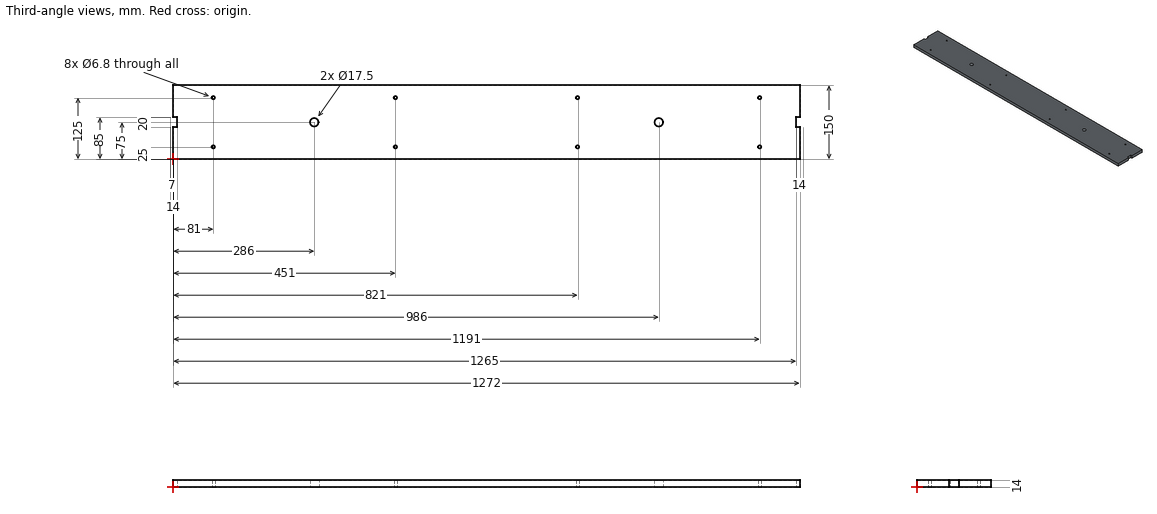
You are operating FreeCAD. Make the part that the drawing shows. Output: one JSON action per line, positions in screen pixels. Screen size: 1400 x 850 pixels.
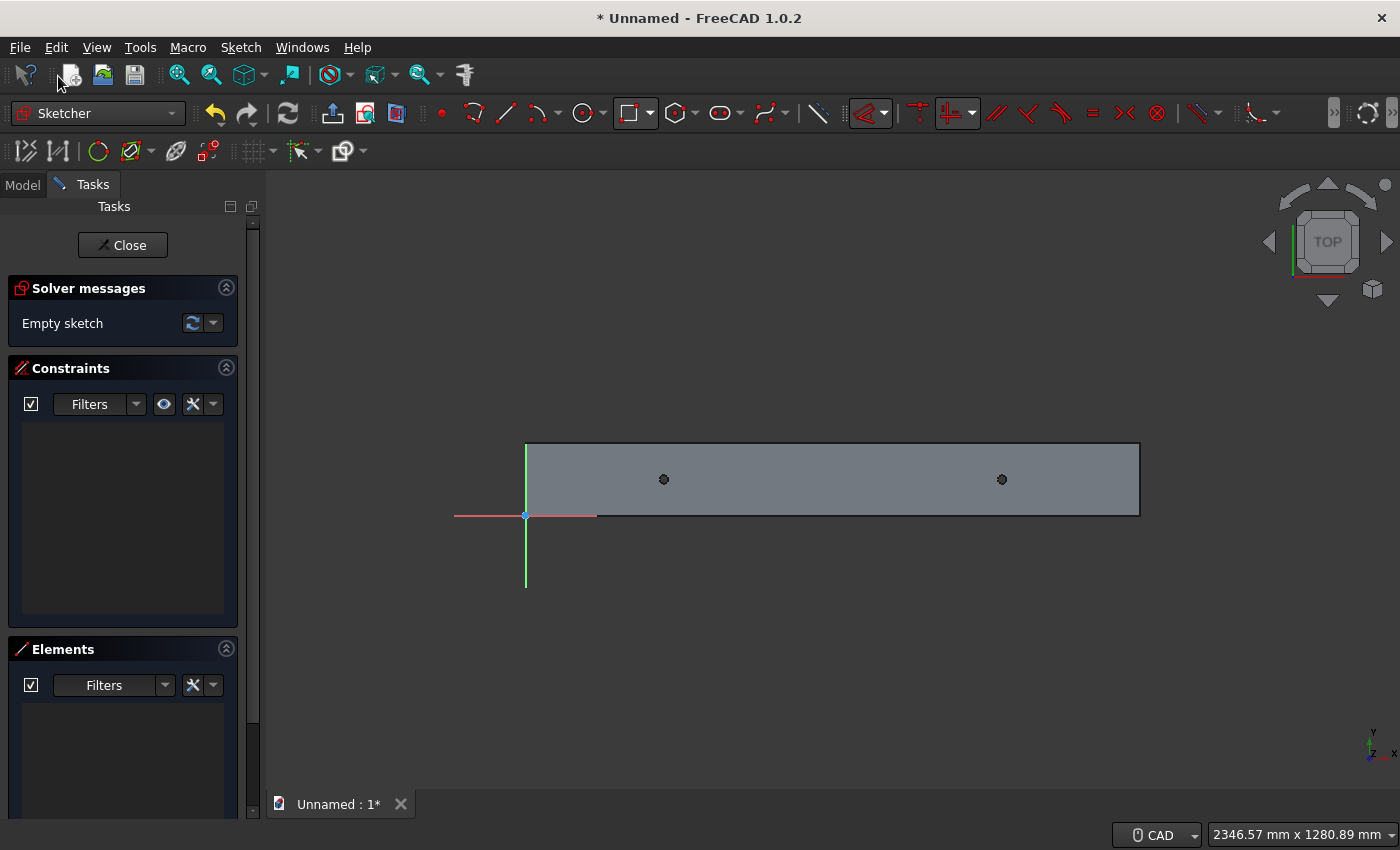
{"action": "left_click", "coordinate": [584, 114]}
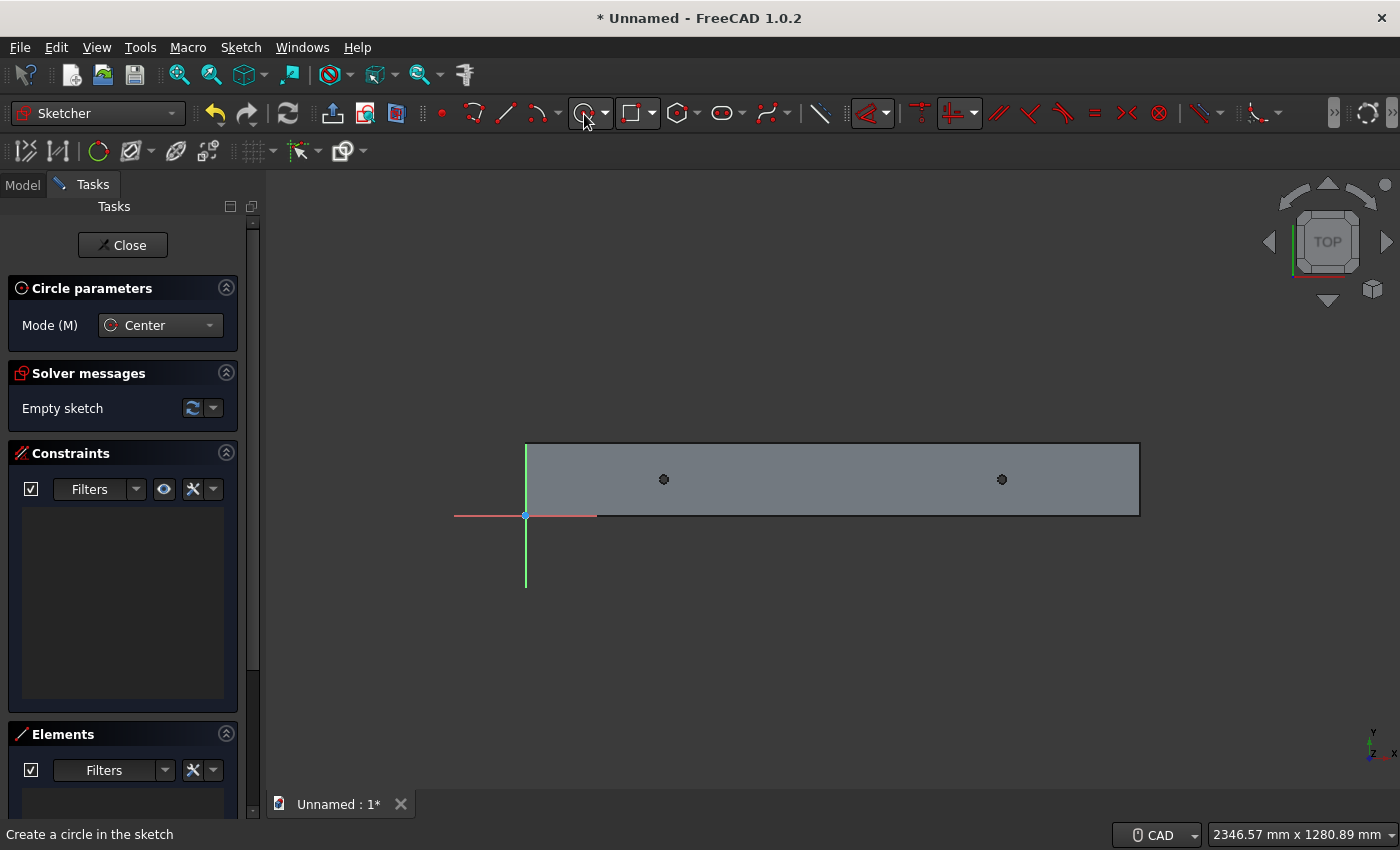
{"action": "scroll", "coordinate": [565, 455], "scroll_direction": "up", "scroll_amount": 14}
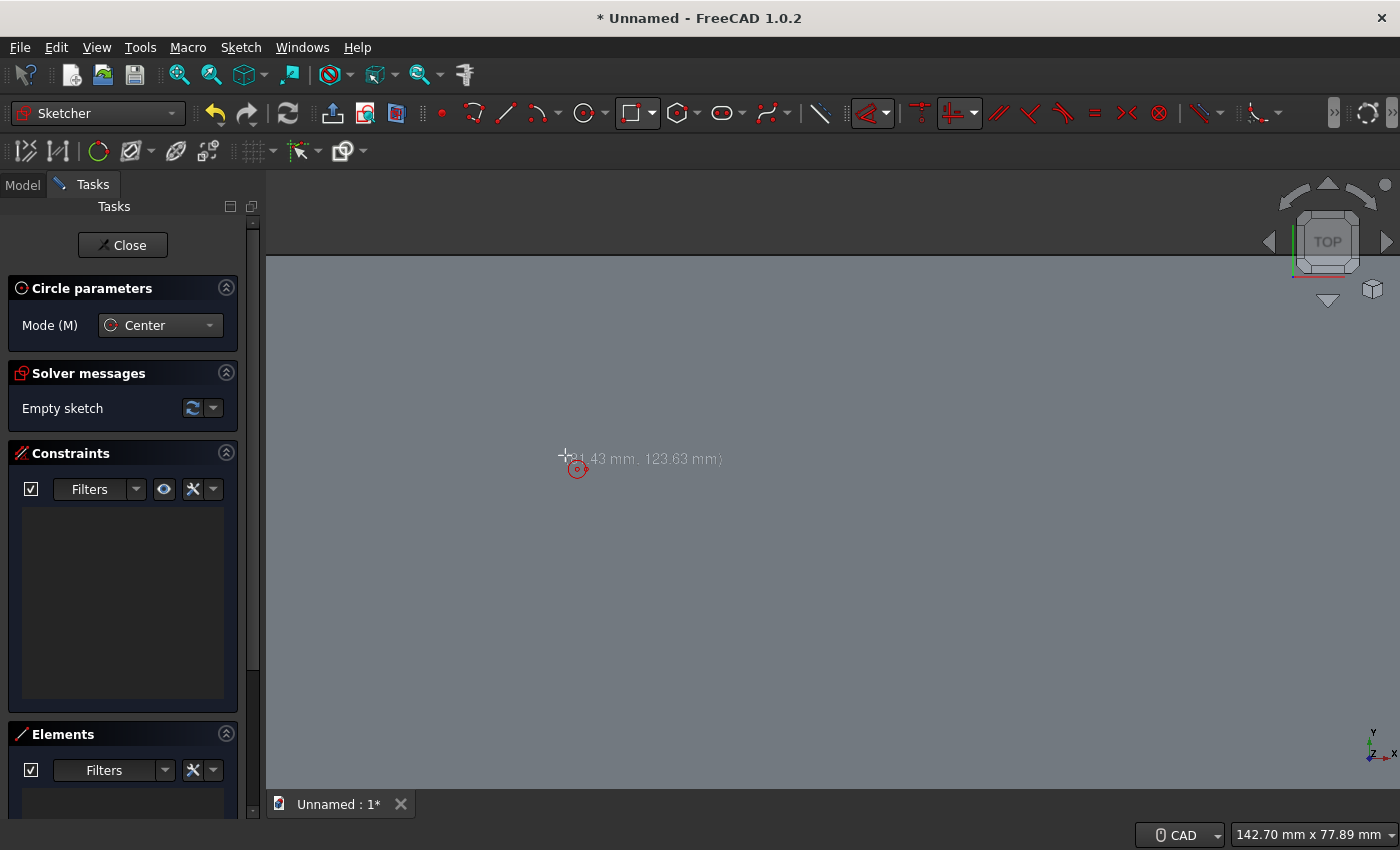
{"action": "scroll", "coordinate": [452, 443], "scroll_direction": "down", "scroll_amount": 13}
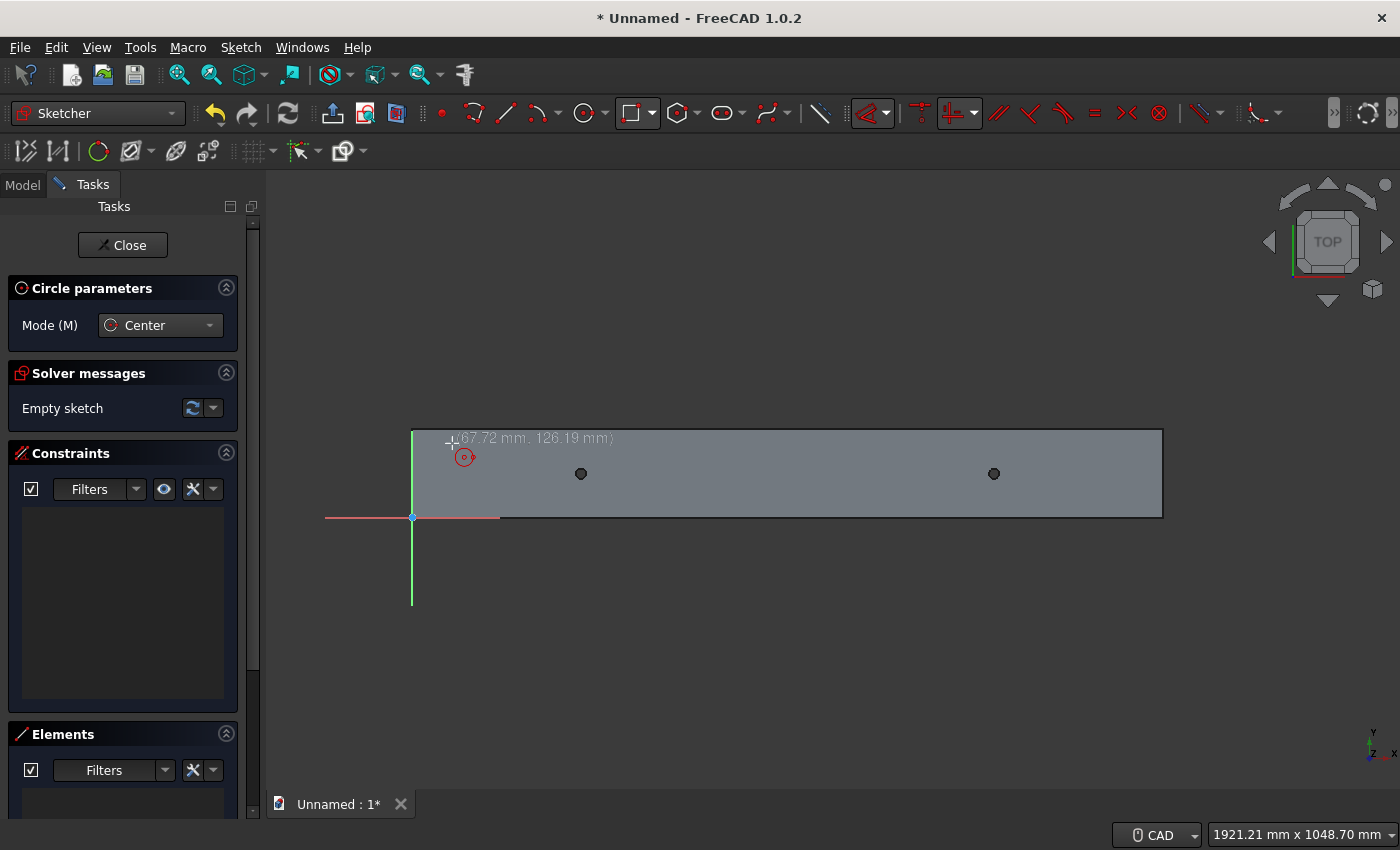
{"action": "left_click", "coordinate": [460, 444]}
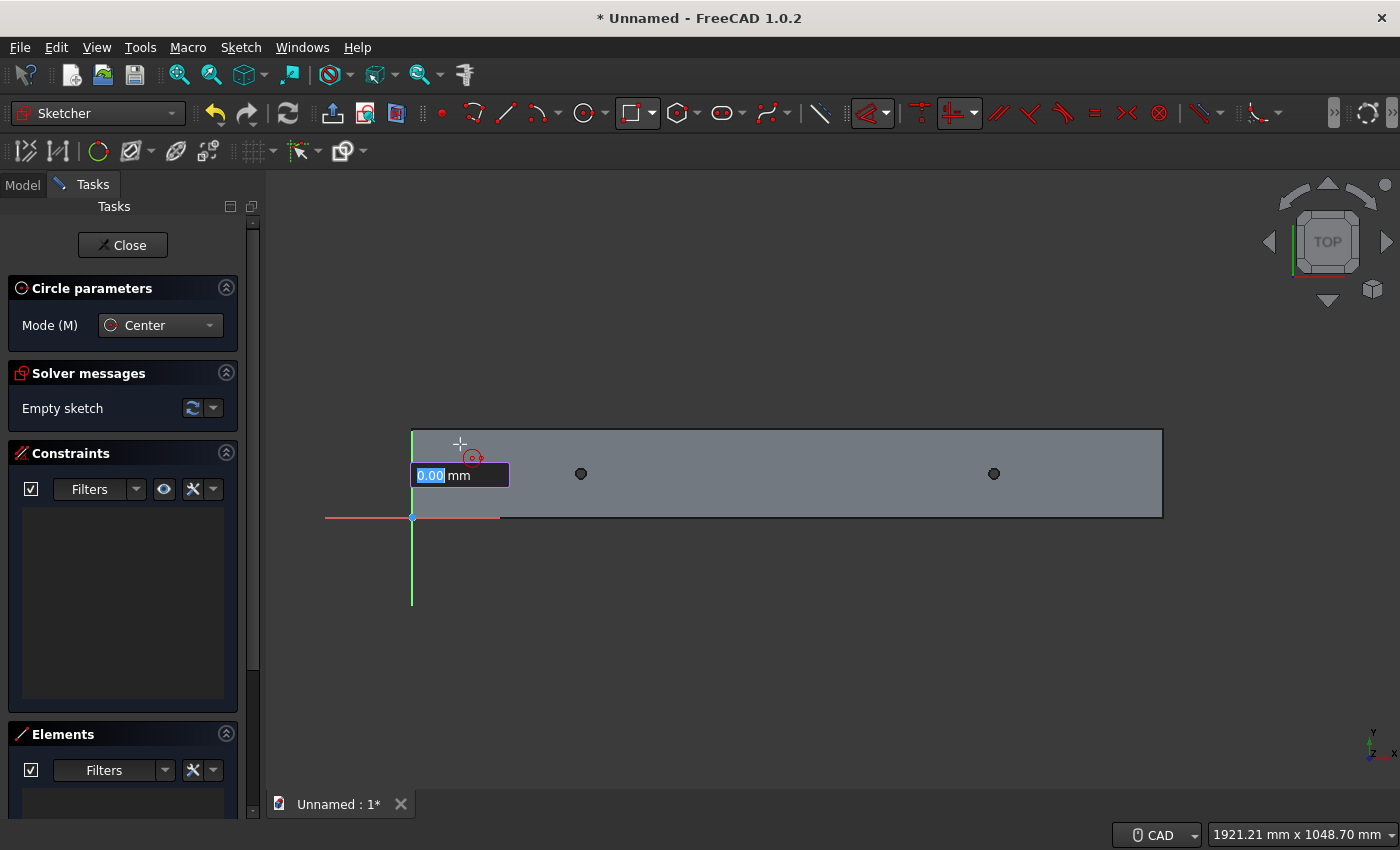
{"action": "scroll", "coordinate": [461, 443], "scroll_direction": "up", "scroll_amount": 11}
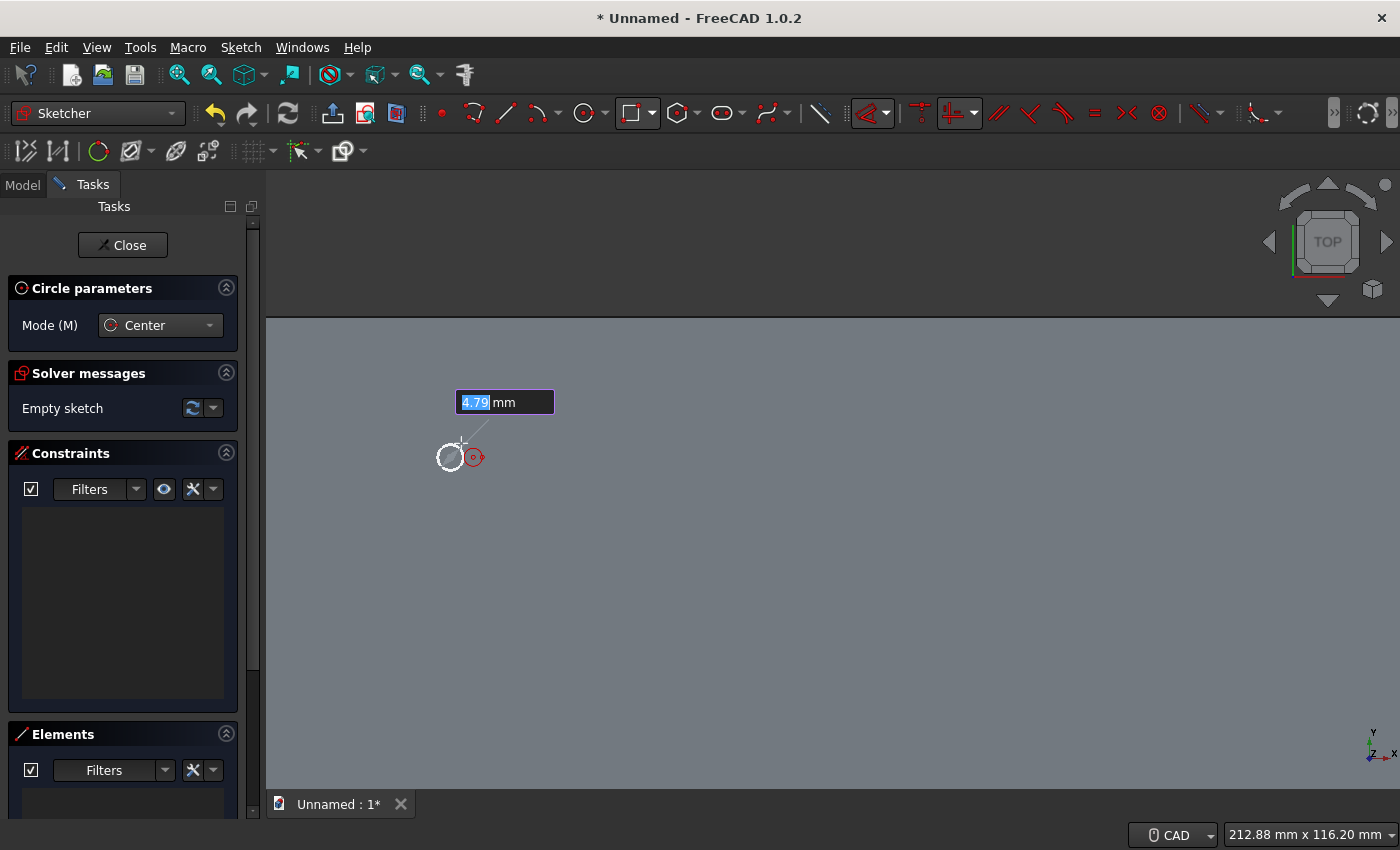
{"action": "left_click", "coordinate": [463, 437]}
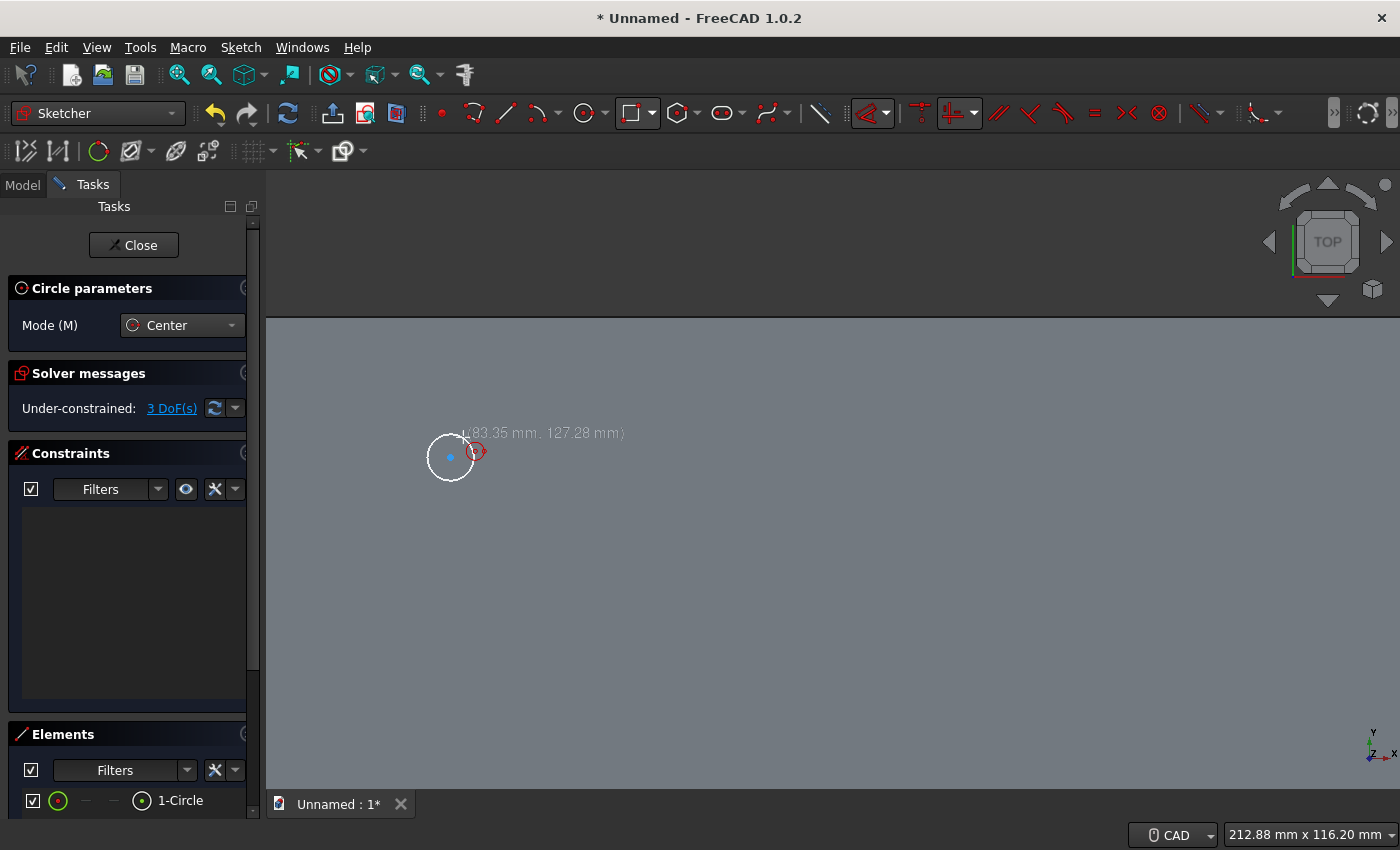
{"action": "scroll", "coordinate": [461, 443], "scroll_direction": "down", "scroll_amount": 11}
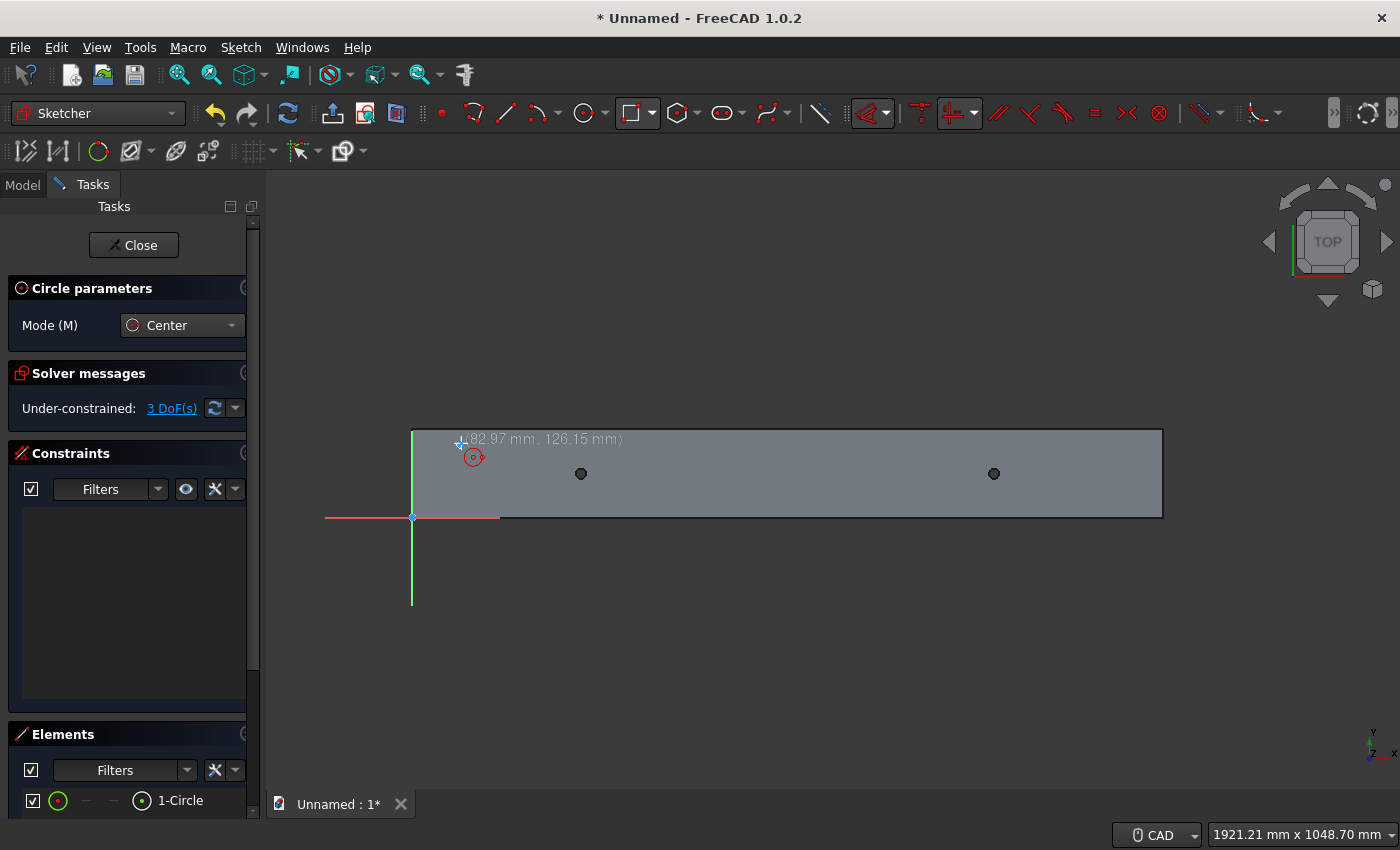
{"action": "scroll", "coordinate": [460, 503], "scroll_direction": "up", "scroll_amount": 13}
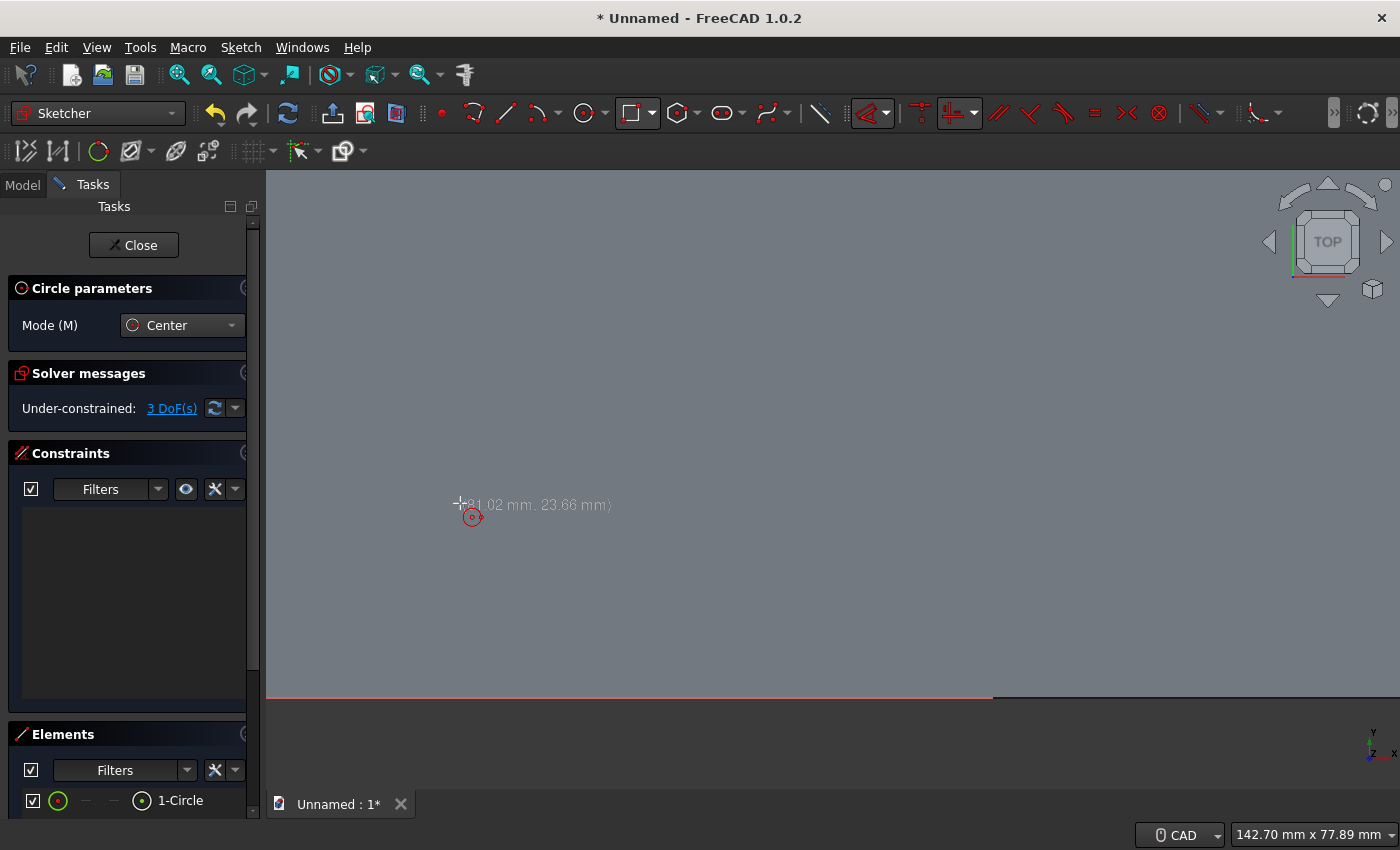
{"action": "scroll", "coordinate": [460, 503], "scroll_direction": "down", "scroll_amount": 13}